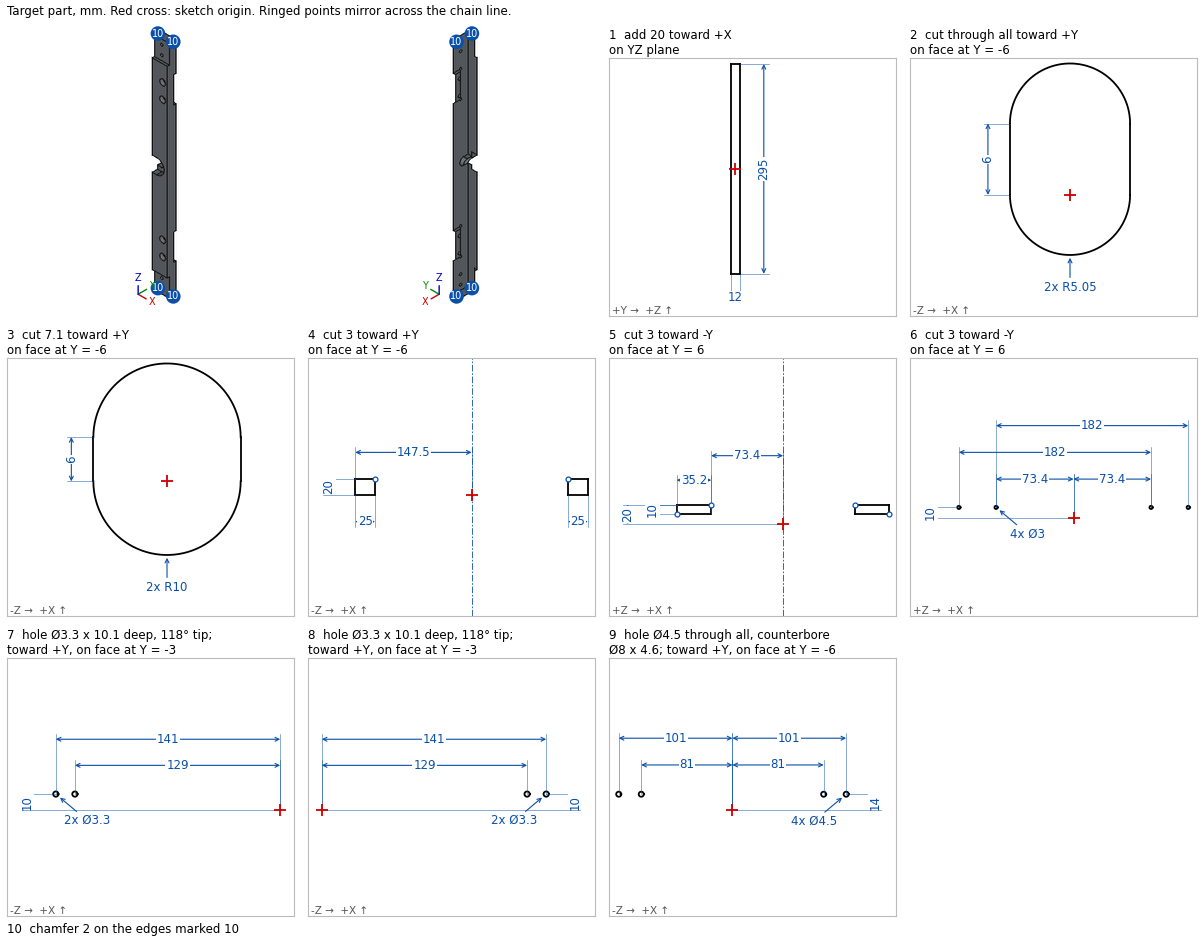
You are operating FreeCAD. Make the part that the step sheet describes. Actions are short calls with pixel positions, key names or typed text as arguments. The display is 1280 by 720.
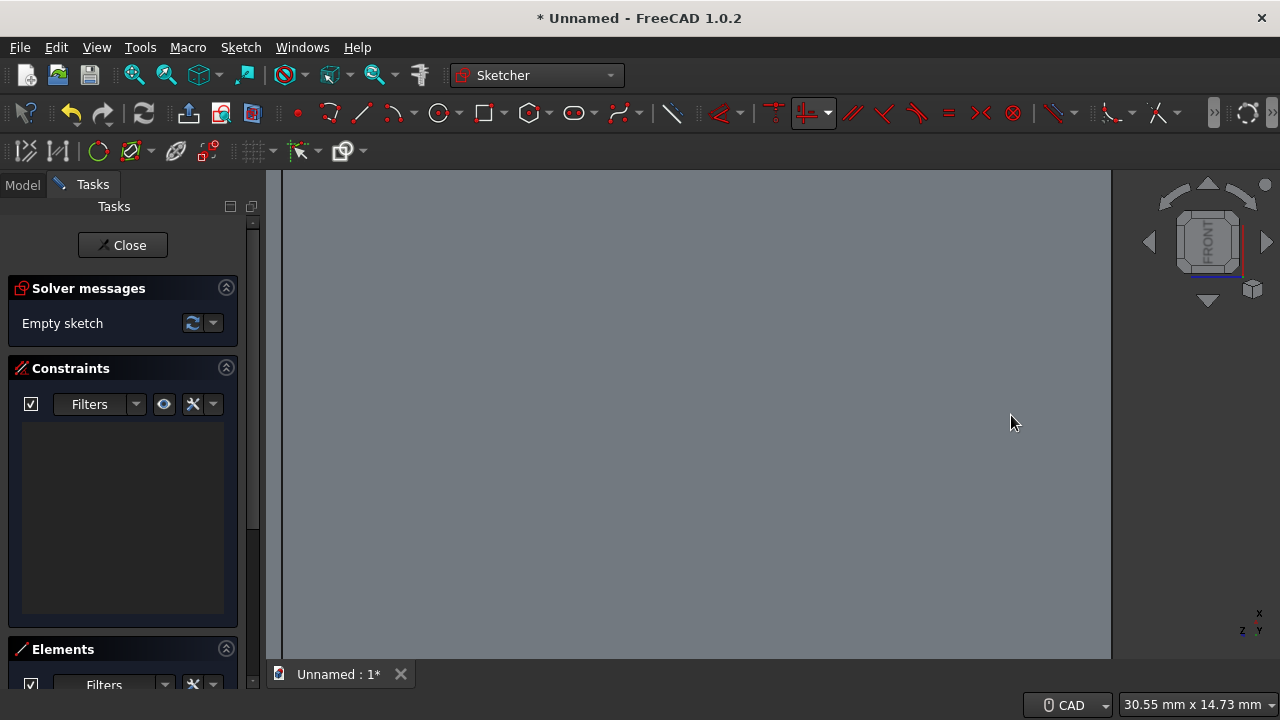
click(440, 114)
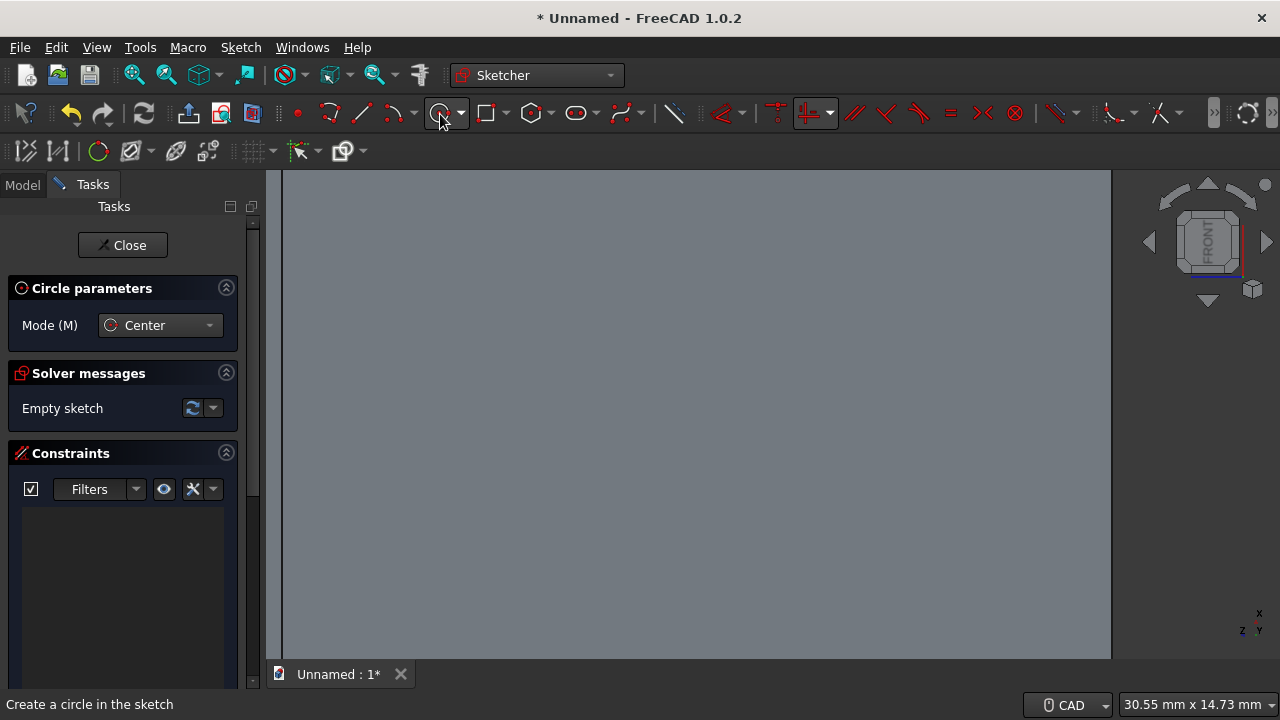
click(897, 395)
click(935, 357)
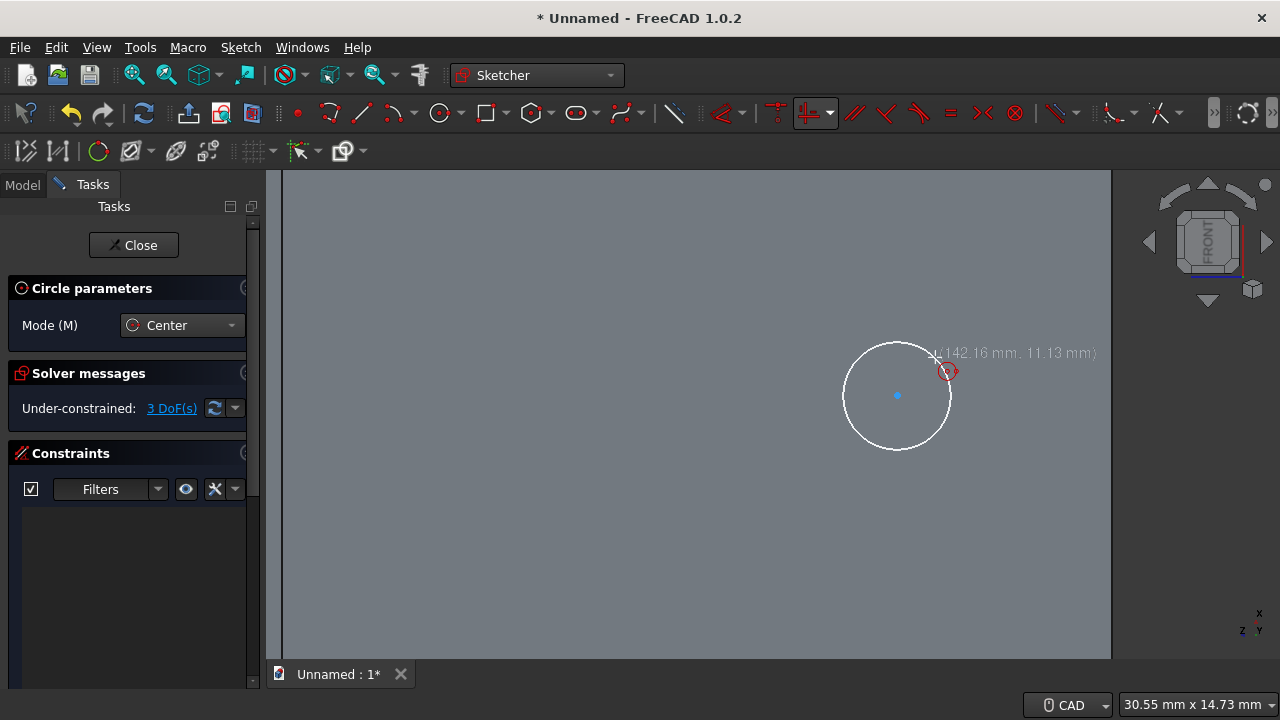
click(498, 395)
click(537, 357)
key(Escape)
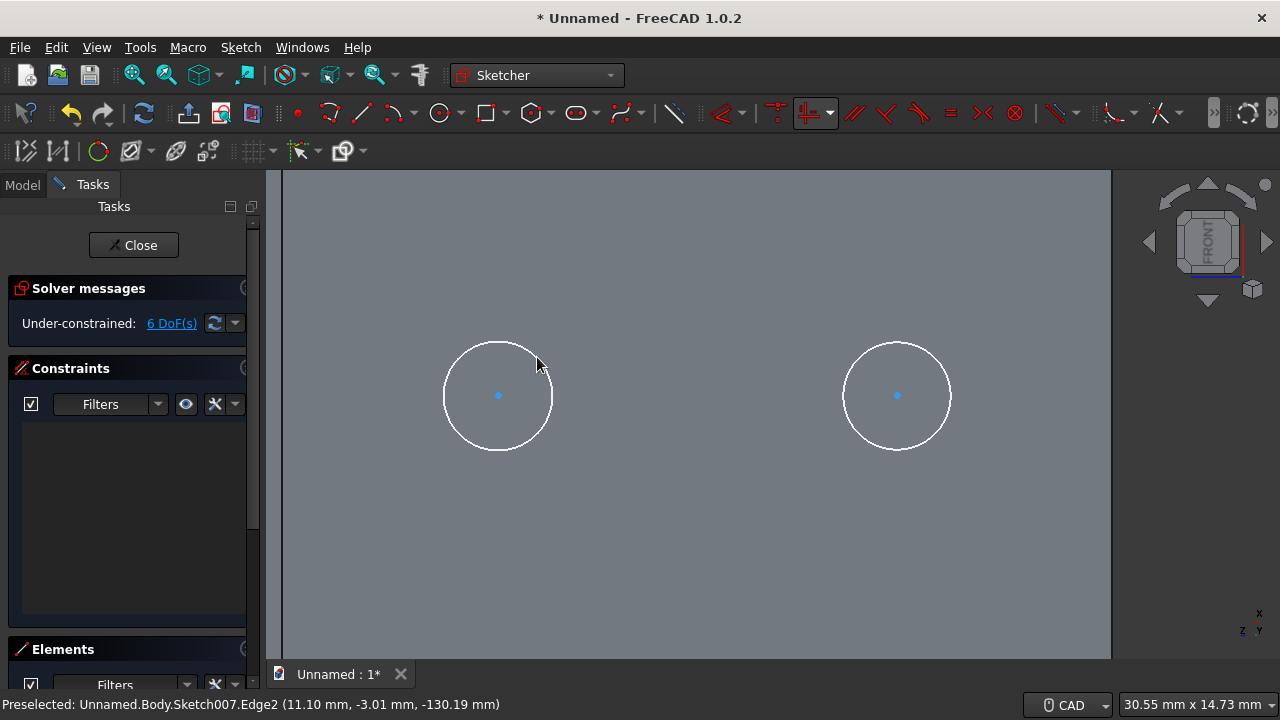
click(935, 358)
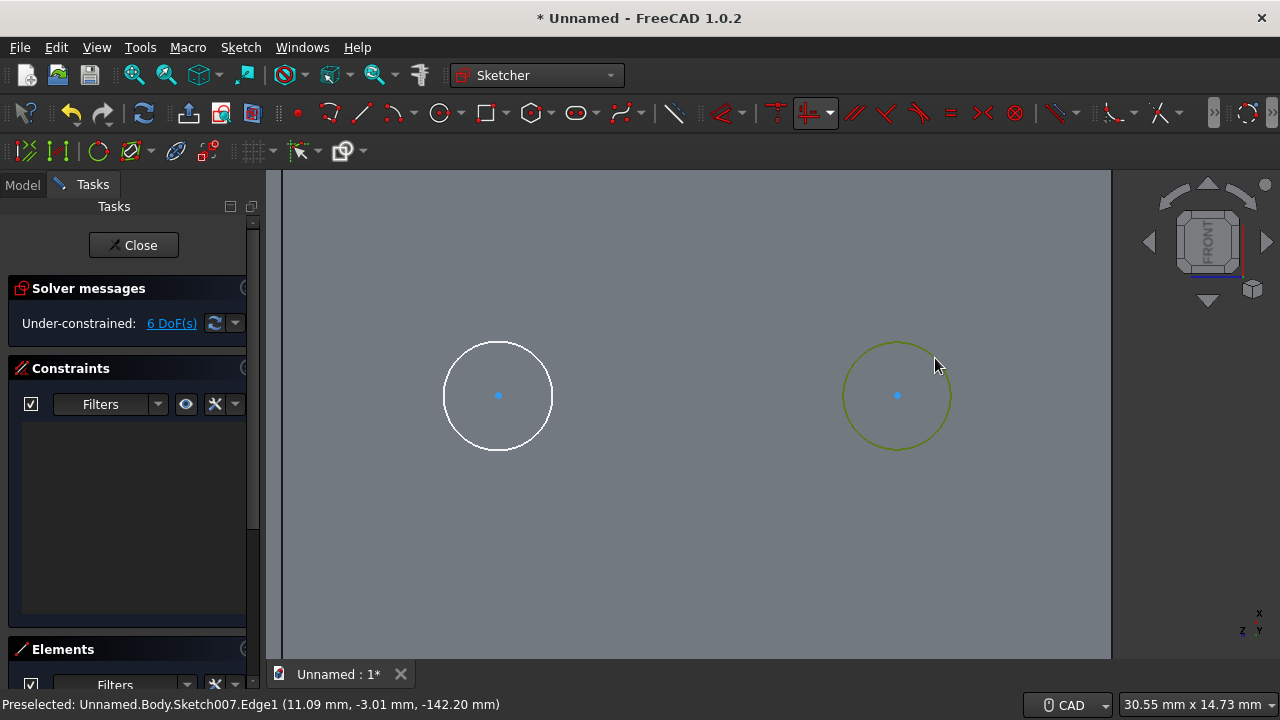
click(536, 357)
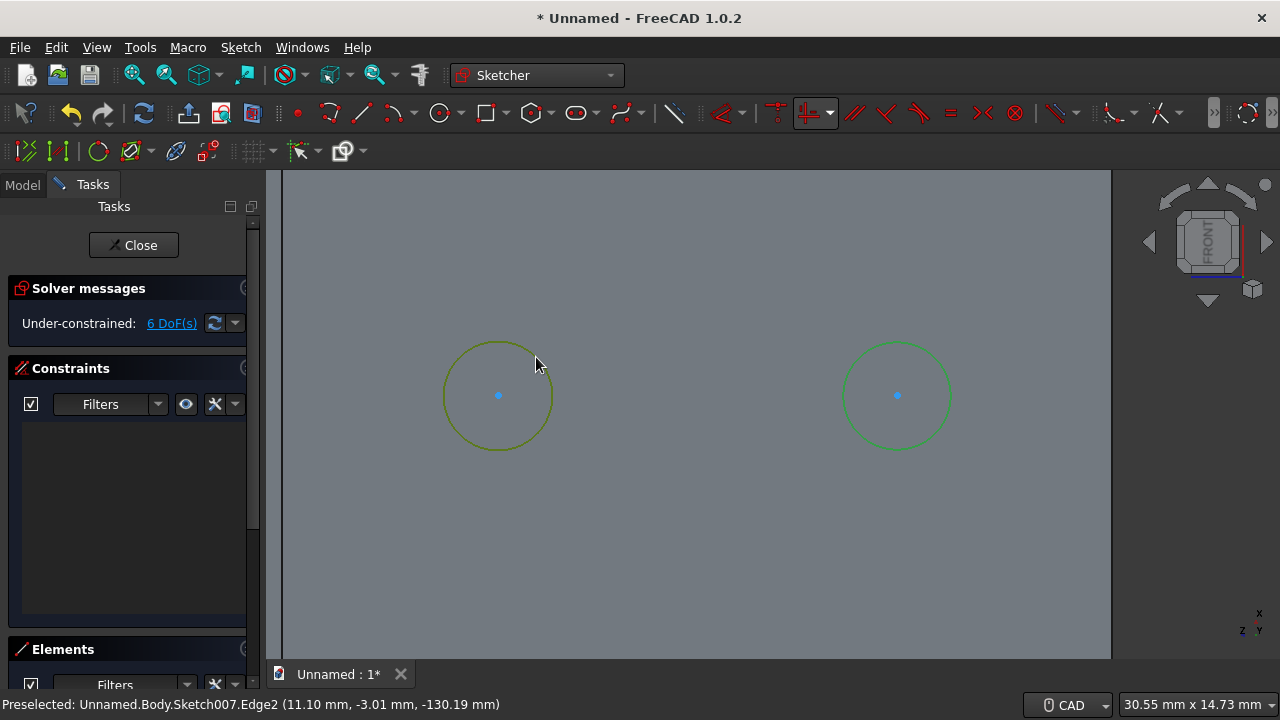
click(952, 114)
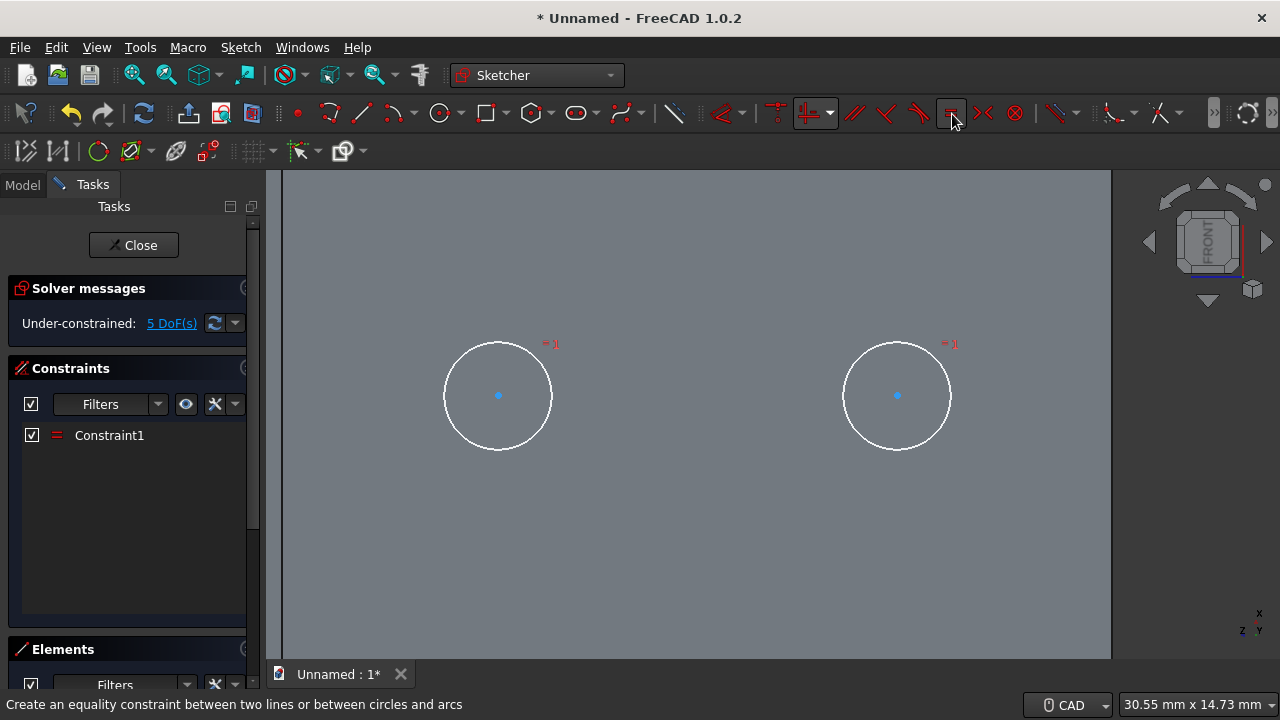
click(897, 396)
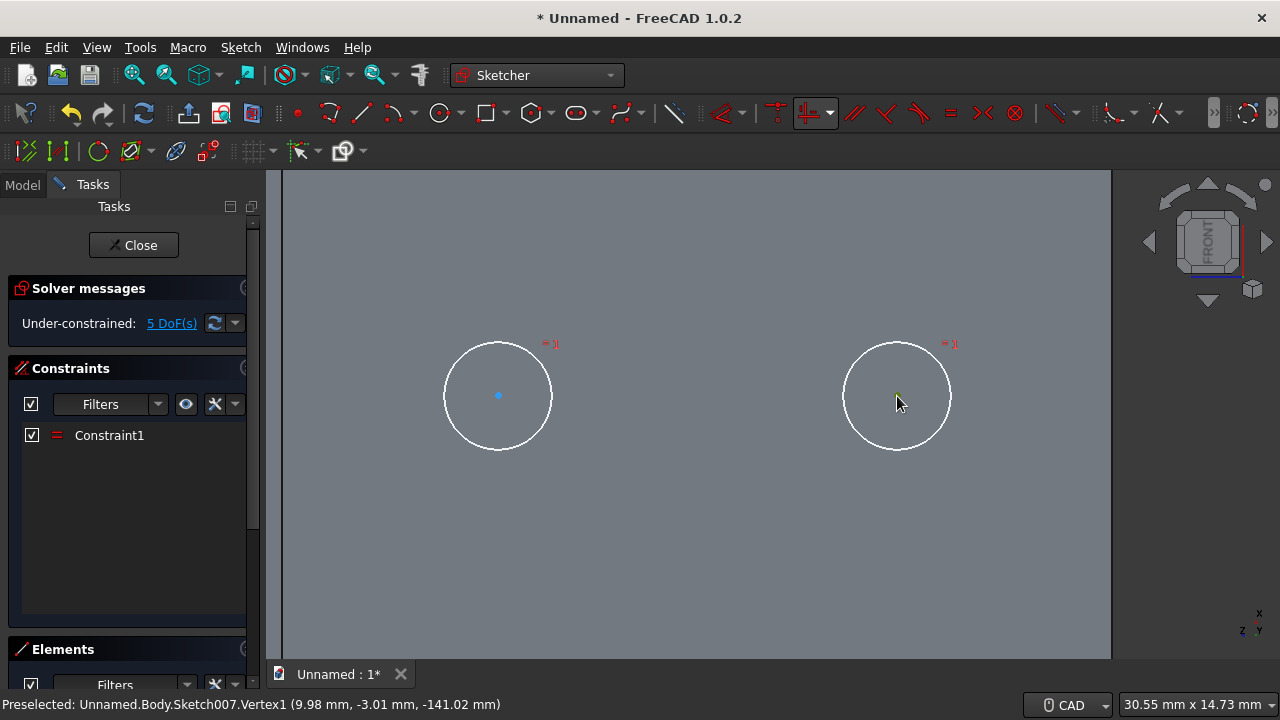
click(498, 396)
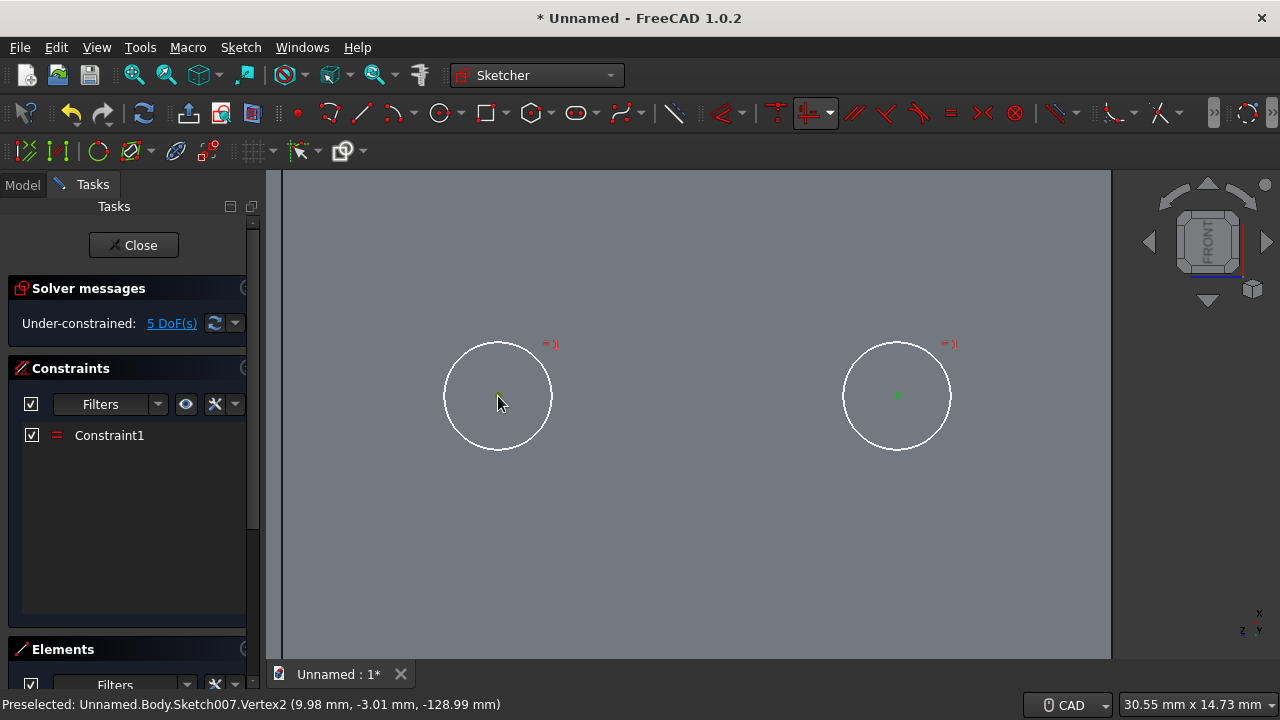
key(h)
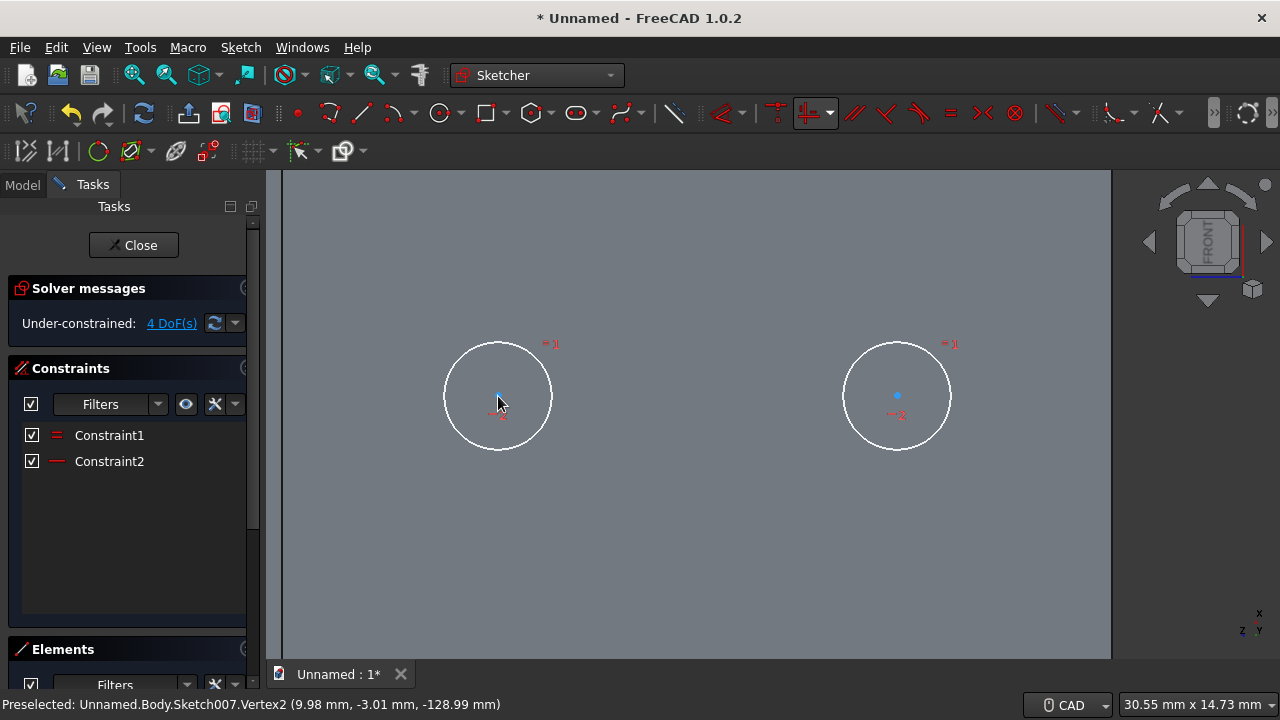
click(722, 114)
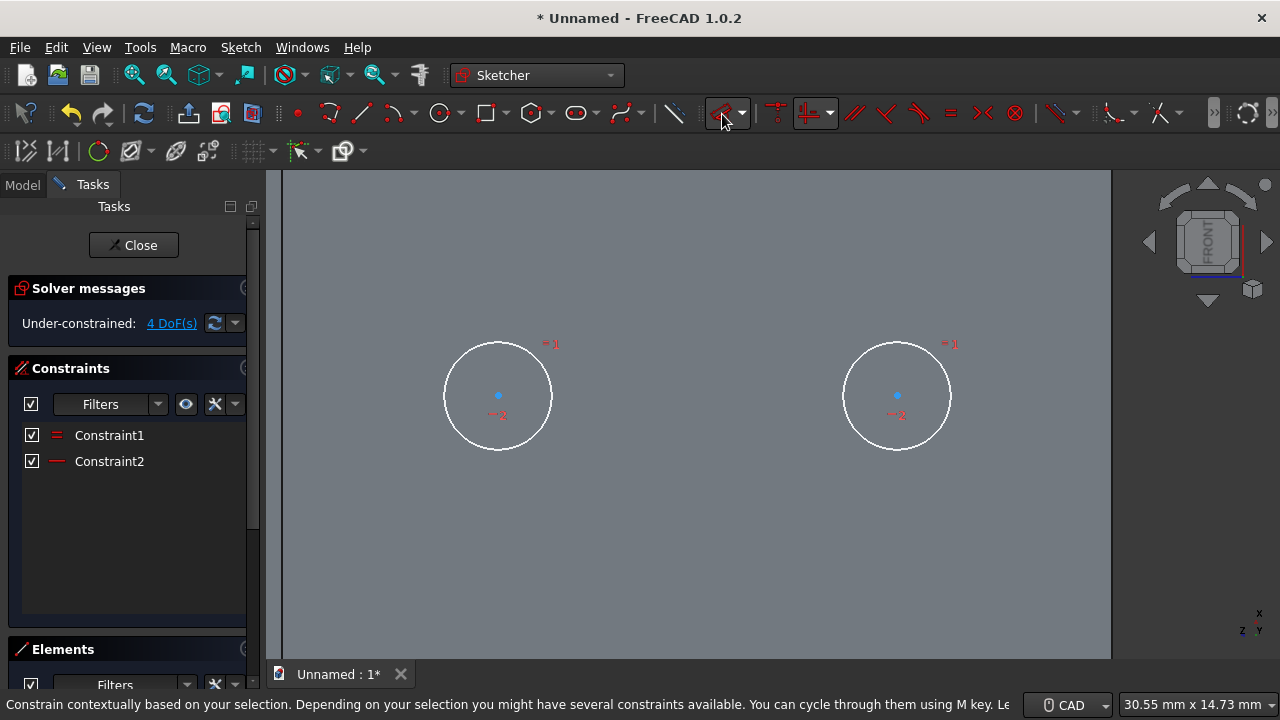
click(935, 358)
click(958, 335)